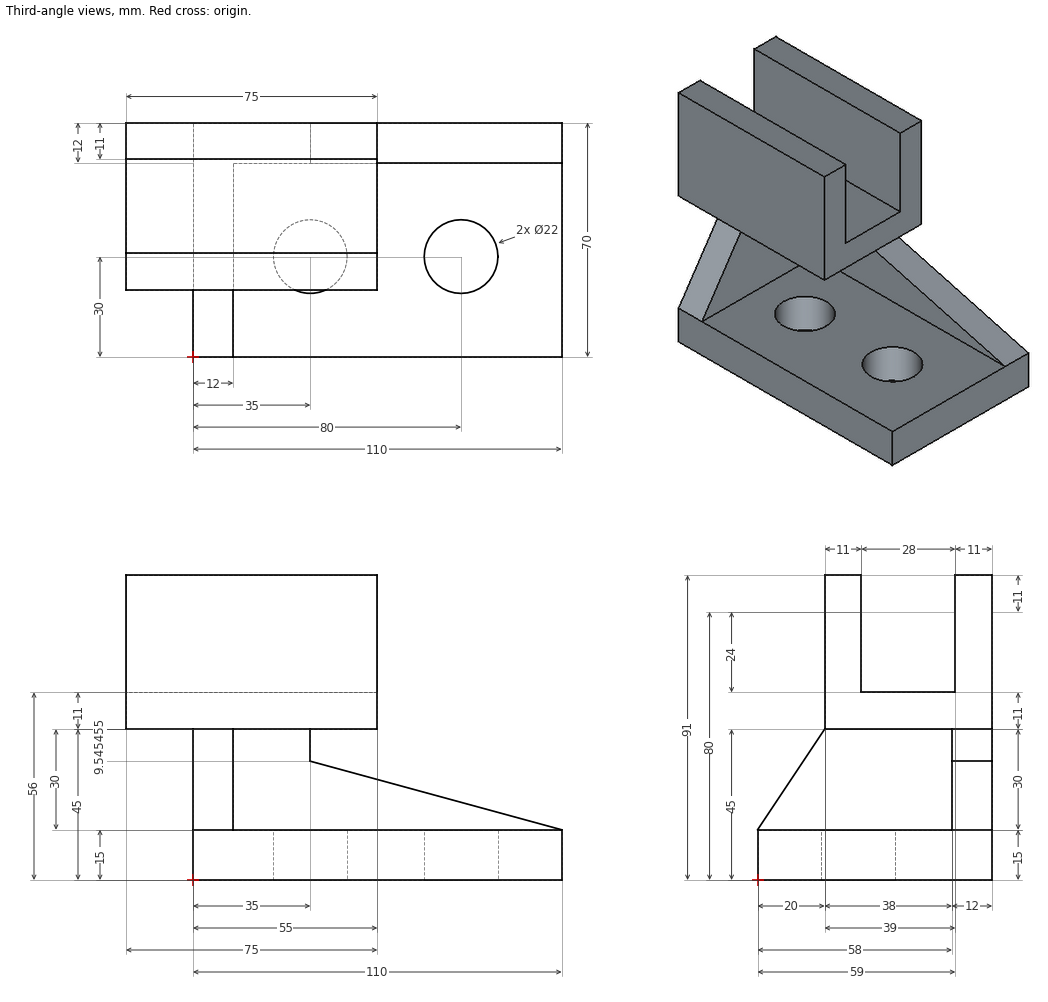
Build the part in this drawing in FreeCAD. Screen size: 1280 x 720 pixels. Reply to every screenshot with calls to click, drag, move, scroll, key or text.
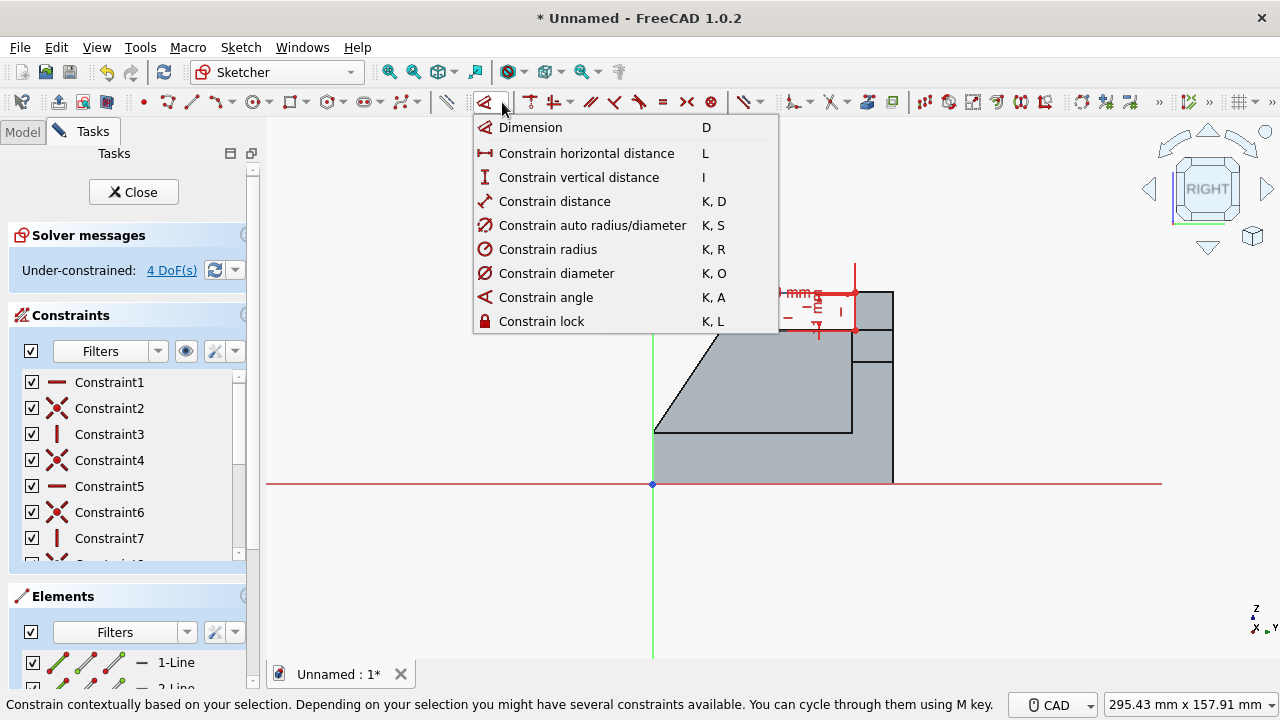
click(626, 153)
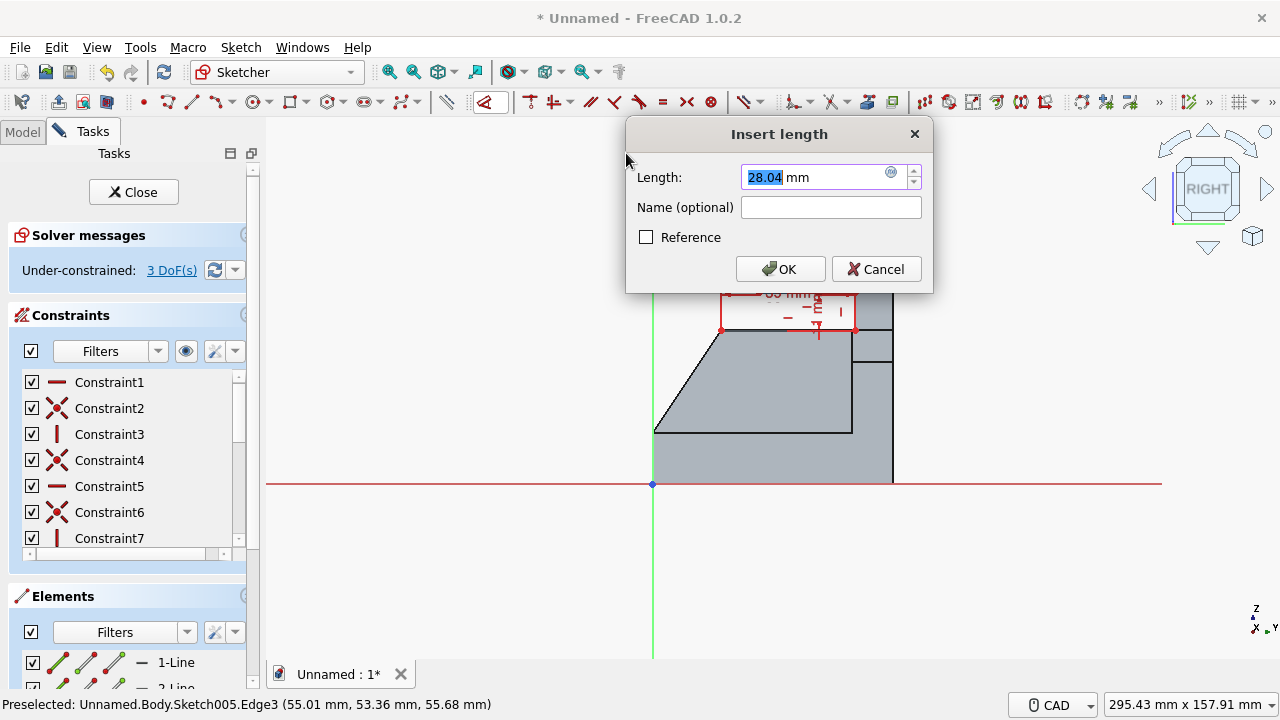
text(28)
key(Return)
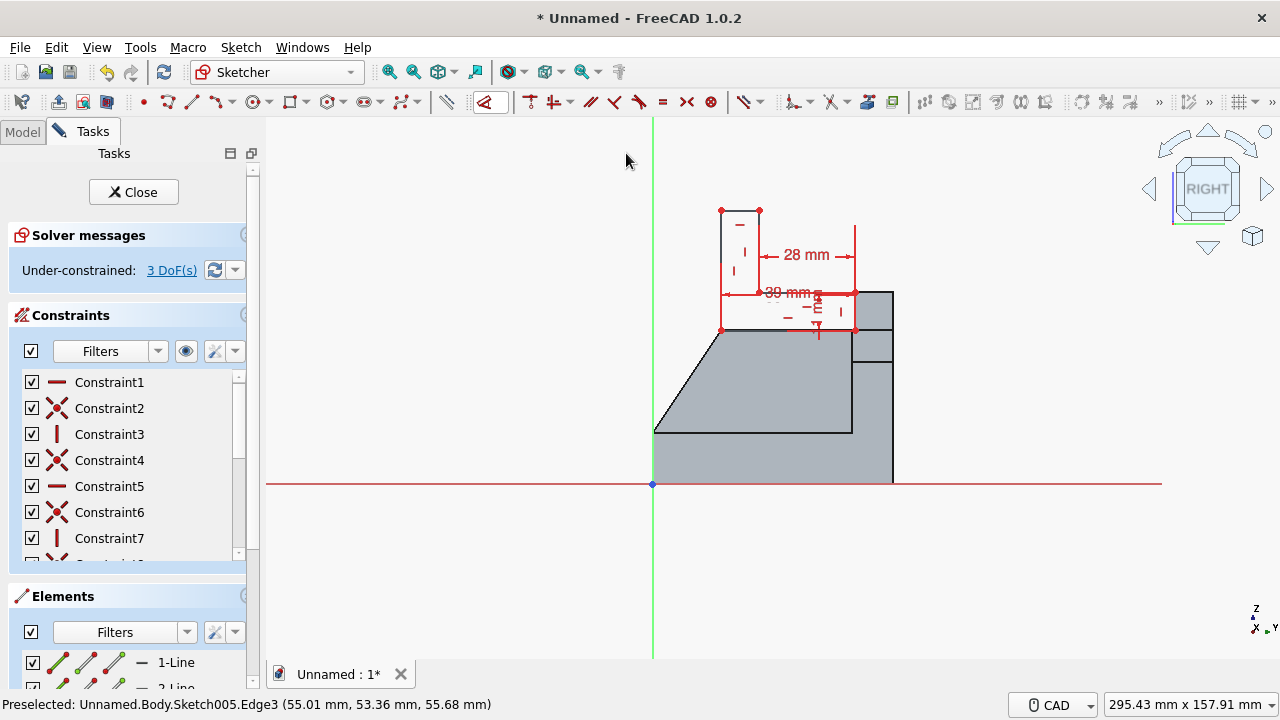
click(759, 268)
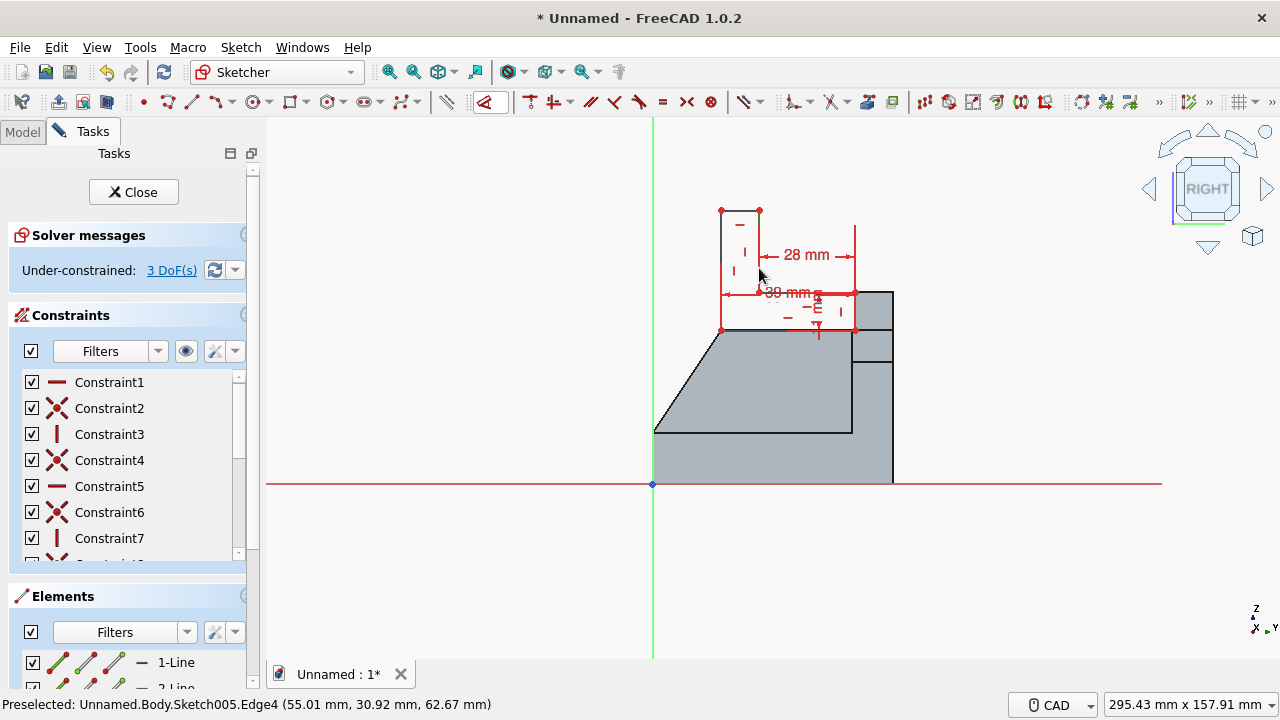
click(502, 102)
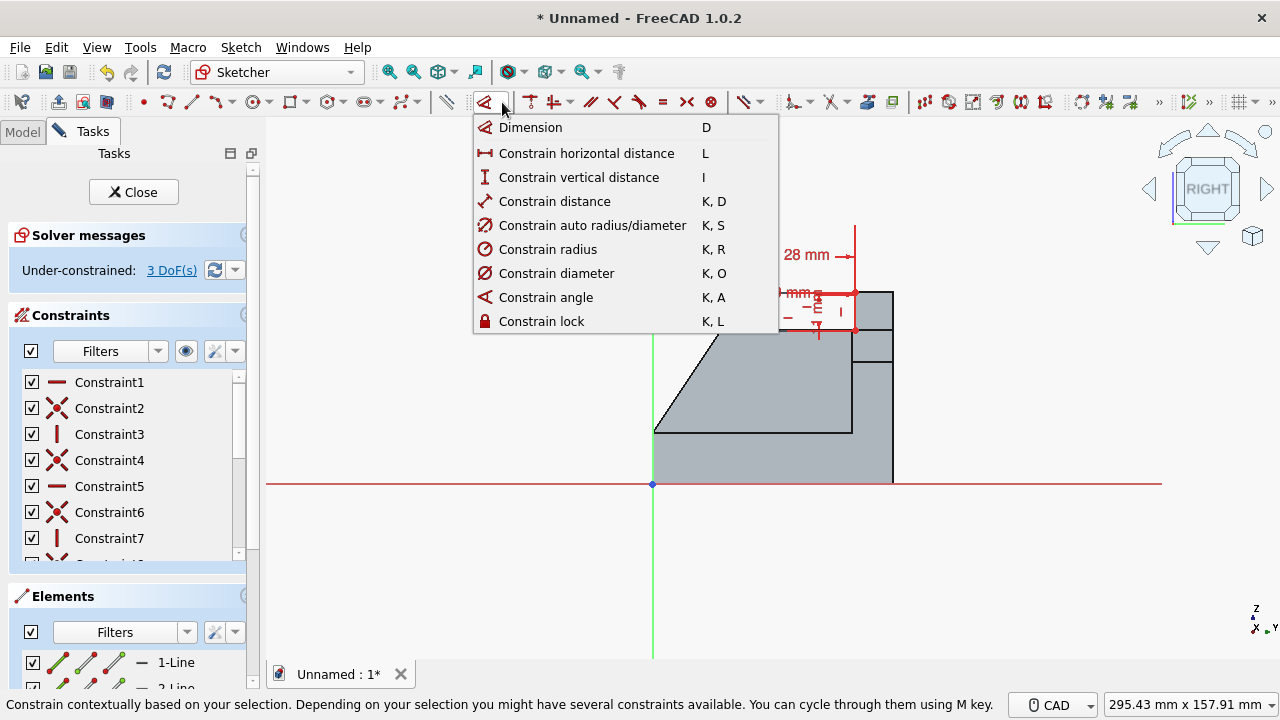
click(626, 177)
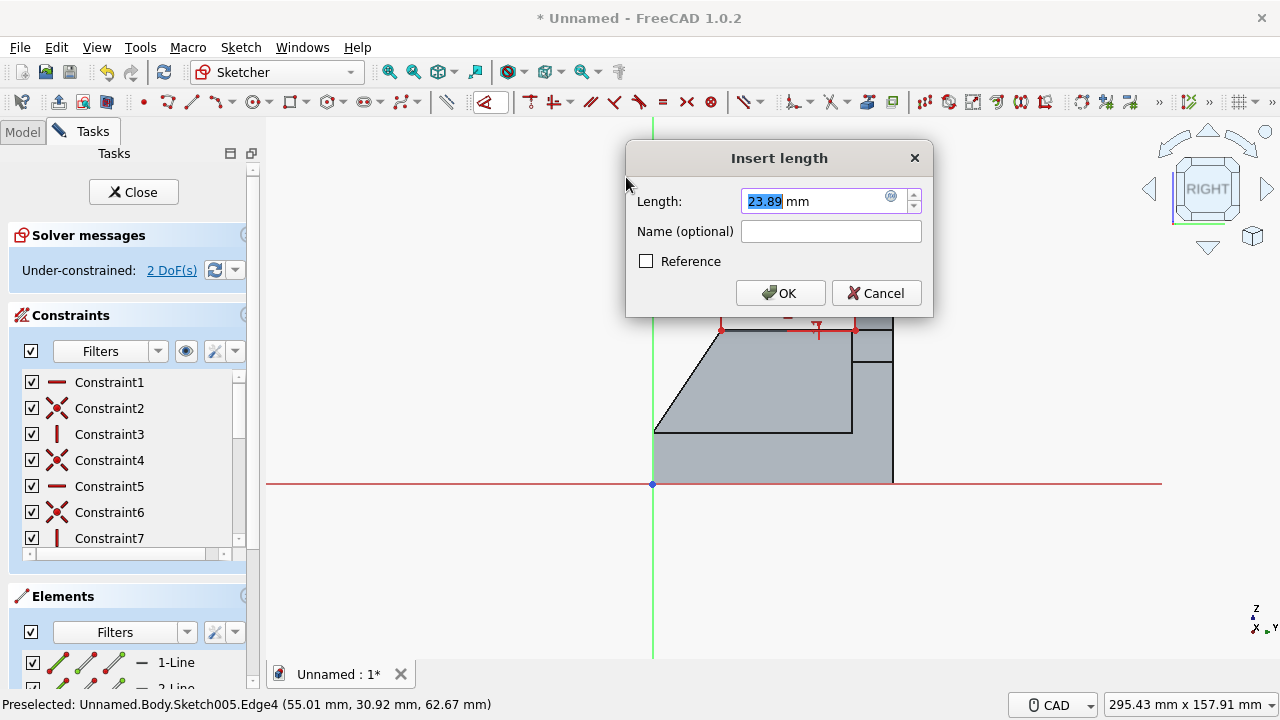
text(24)
key(Return)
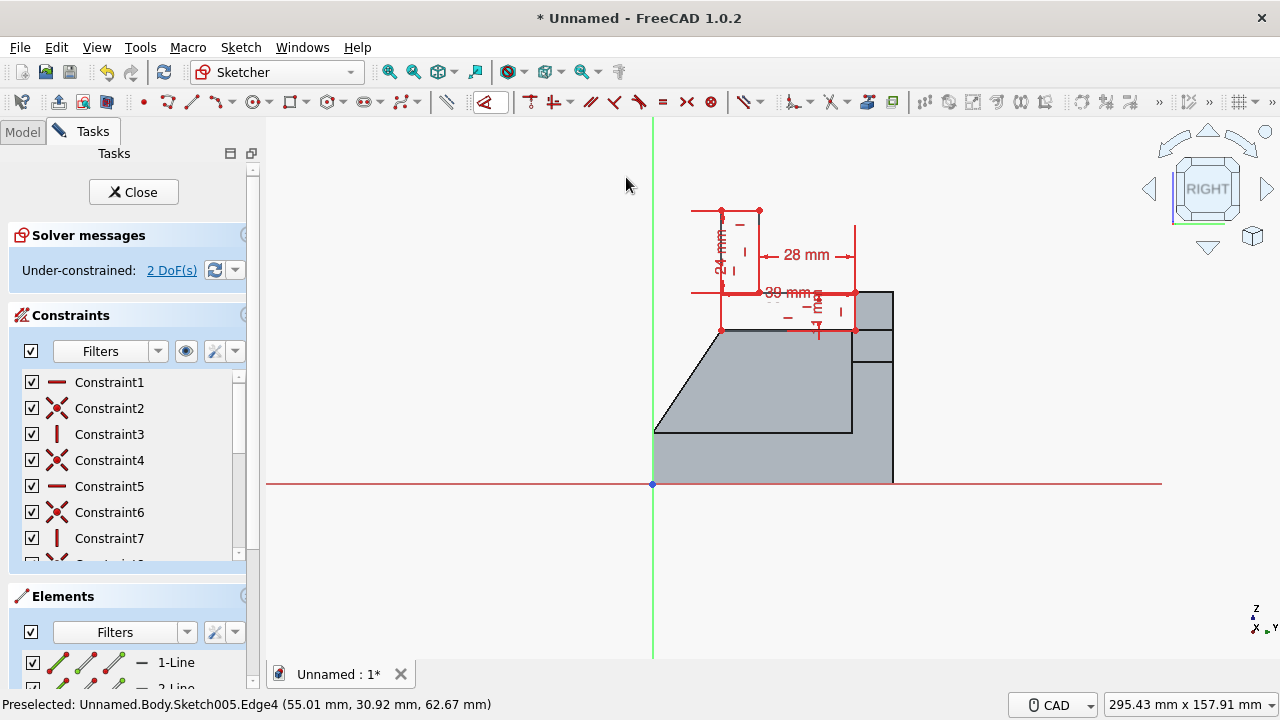
click(721, 331)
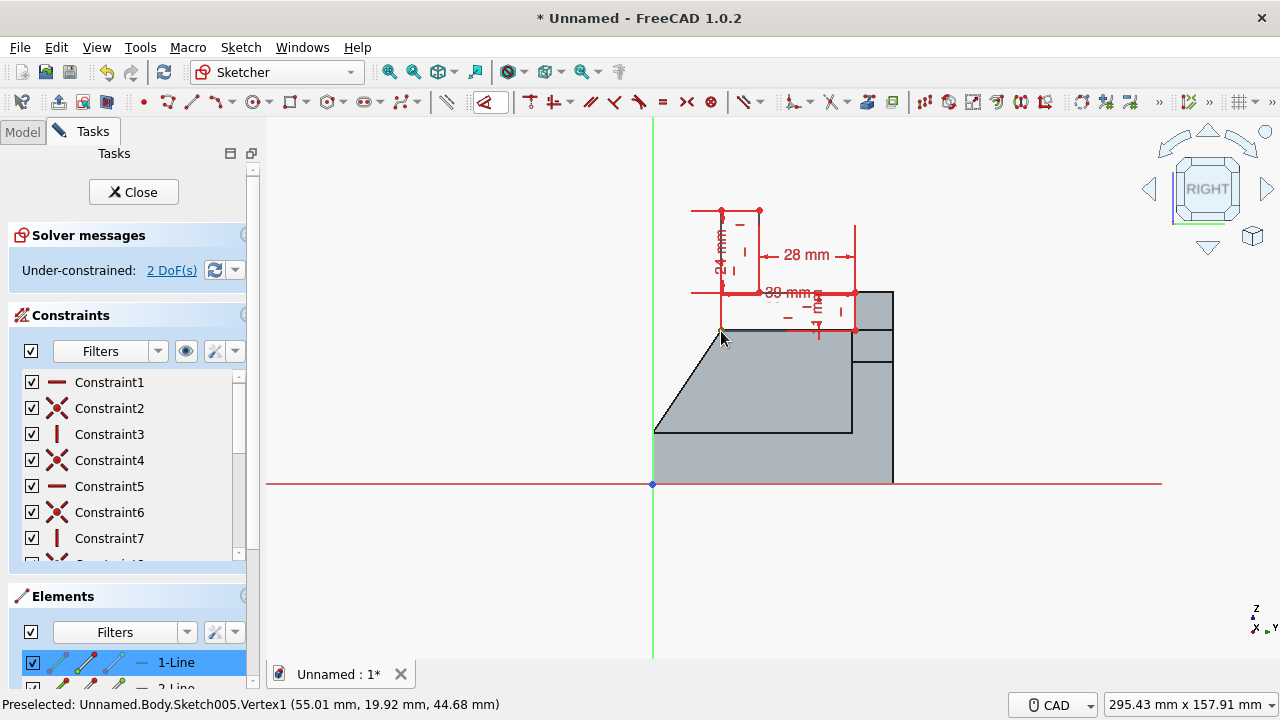
click(502, 102)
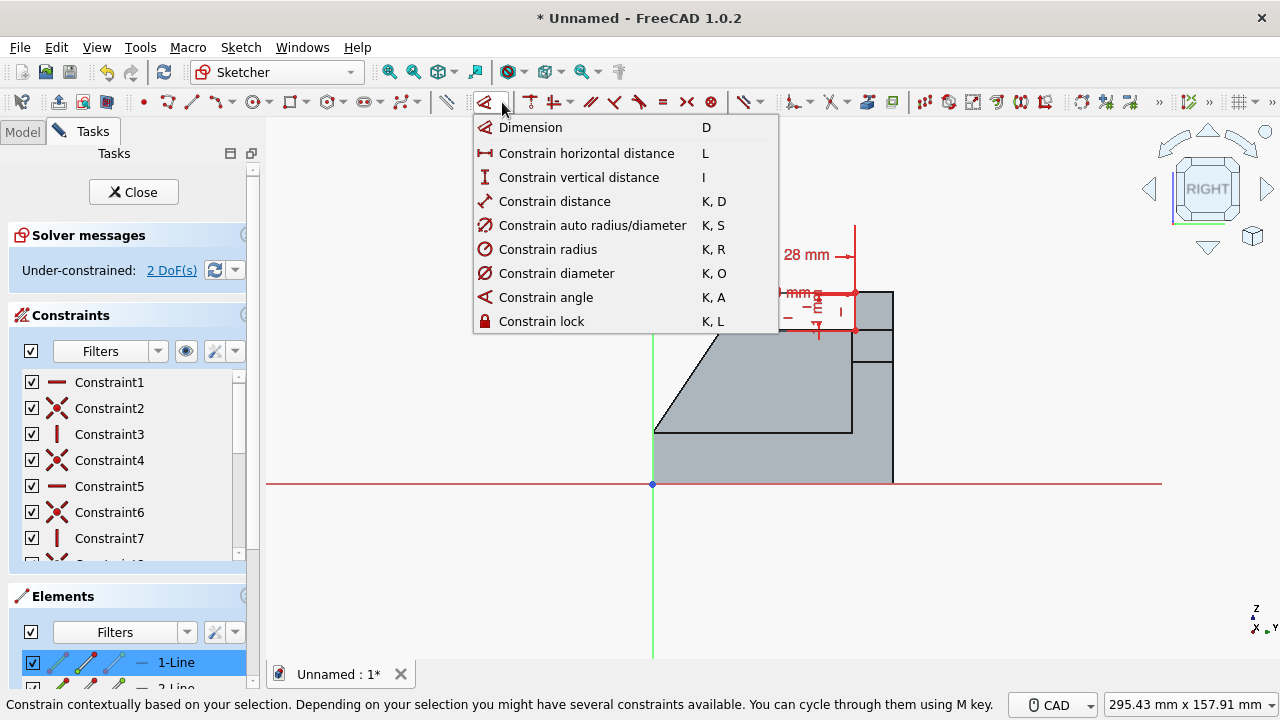
click(626, 153)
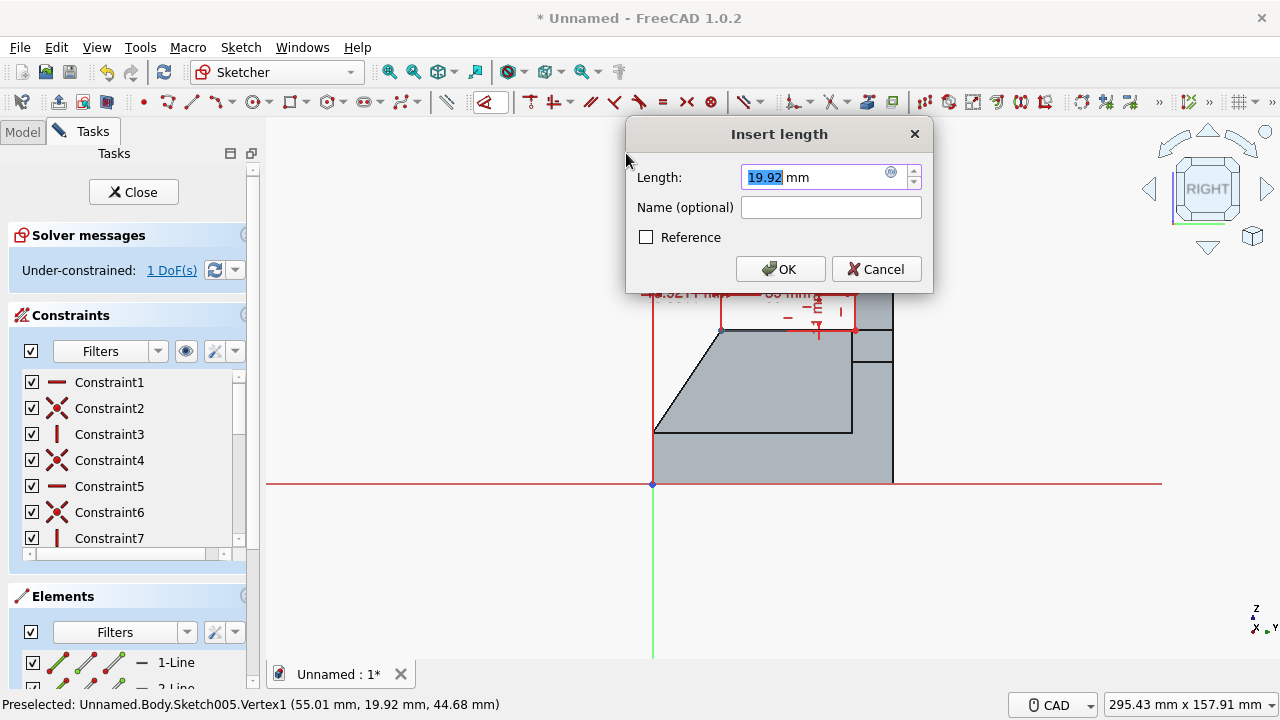
text(20)
key(Return)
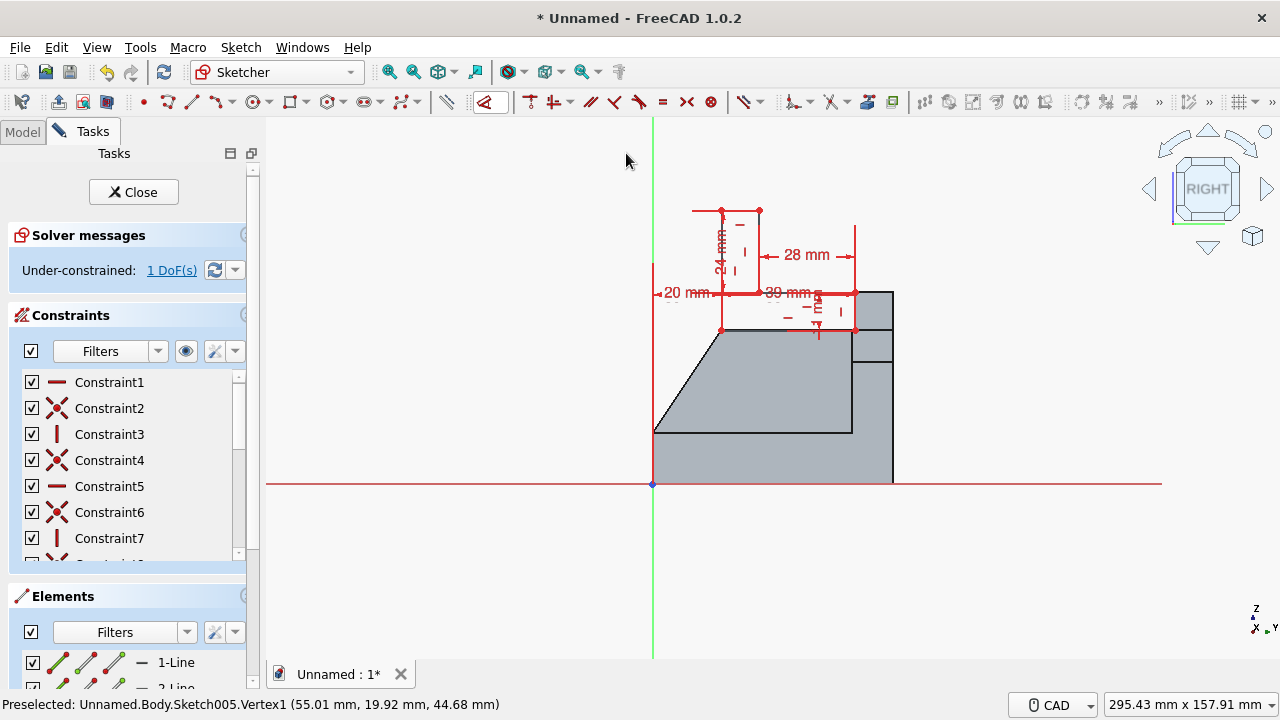
click(722, 331)